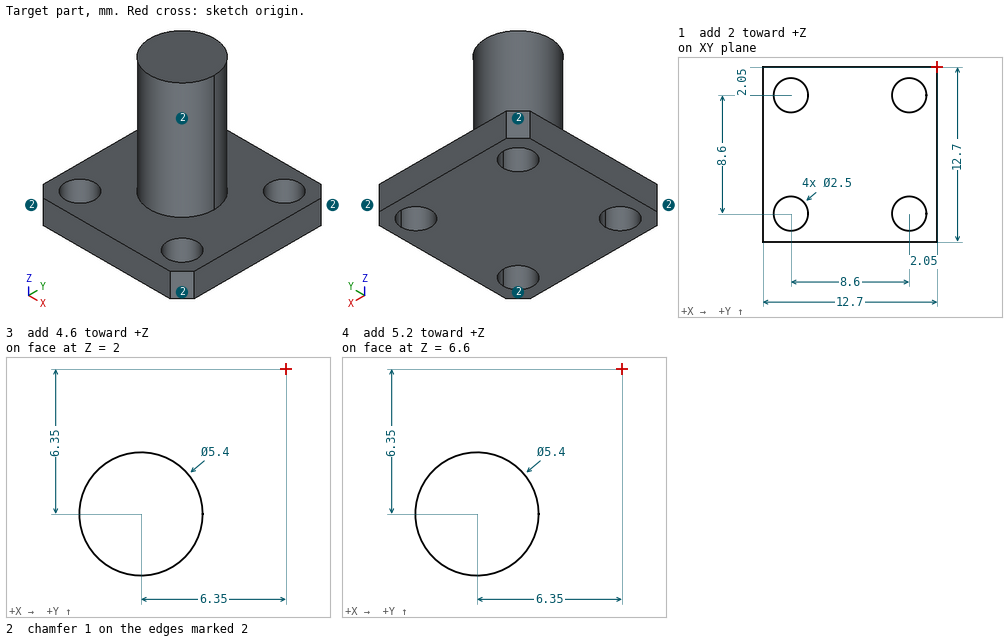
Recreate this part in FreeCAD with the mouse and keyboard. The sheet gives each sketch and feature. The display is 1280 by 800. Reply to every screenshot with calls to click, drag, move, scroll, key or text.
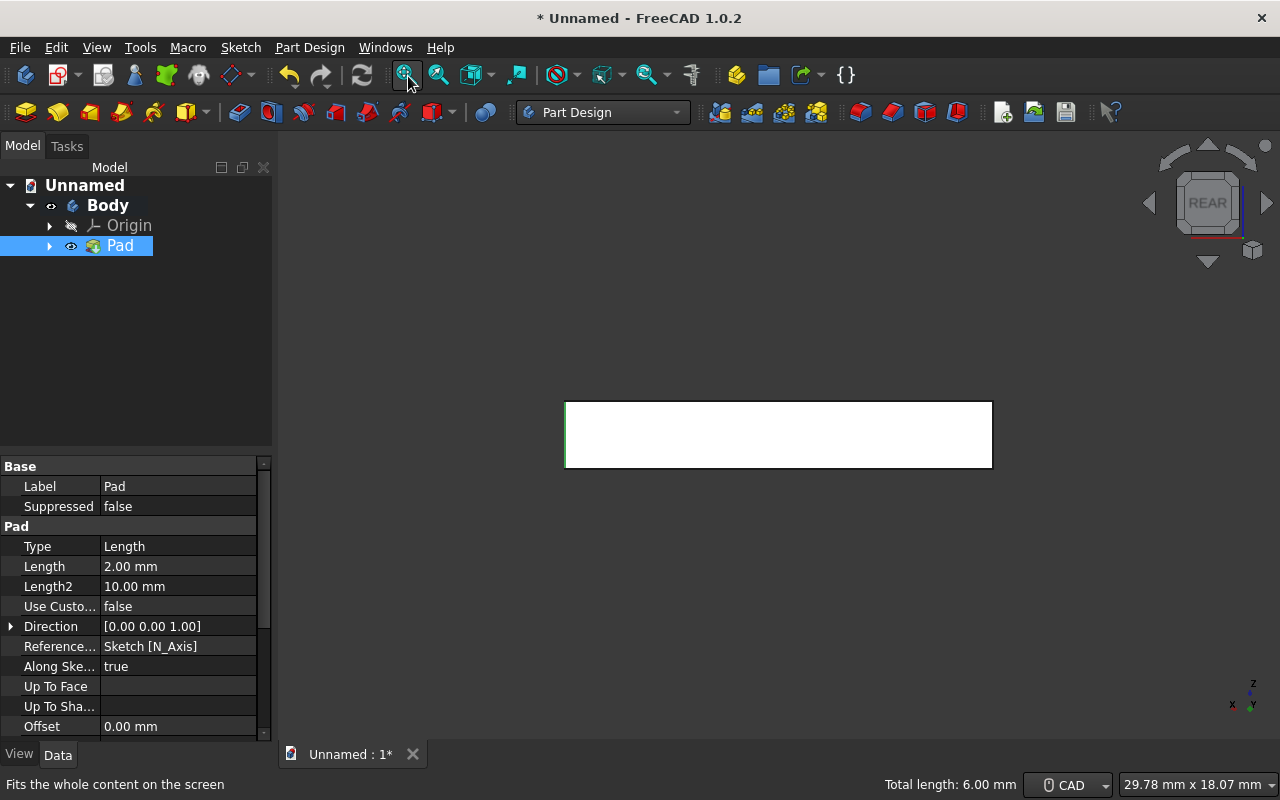
click(993, 434, ctrl)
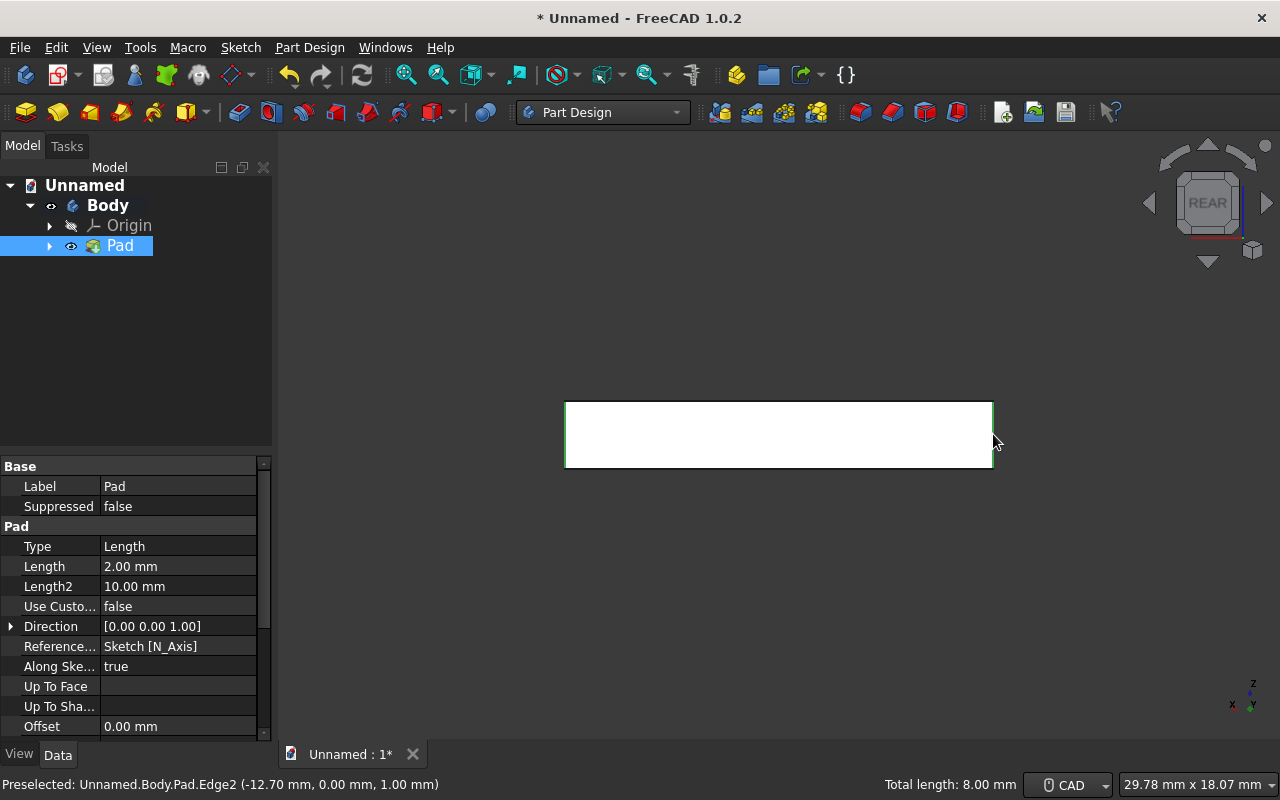
click(894, 112)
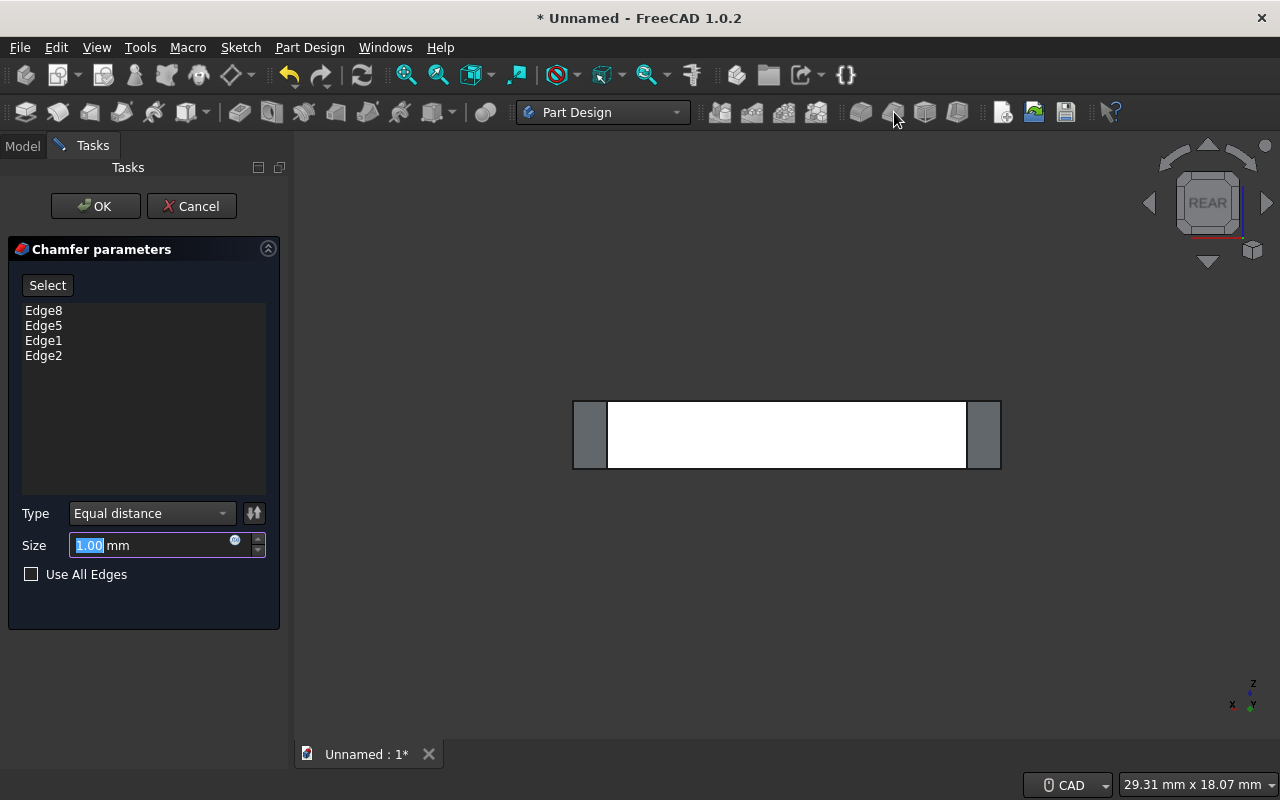
text(1)
key(Tab)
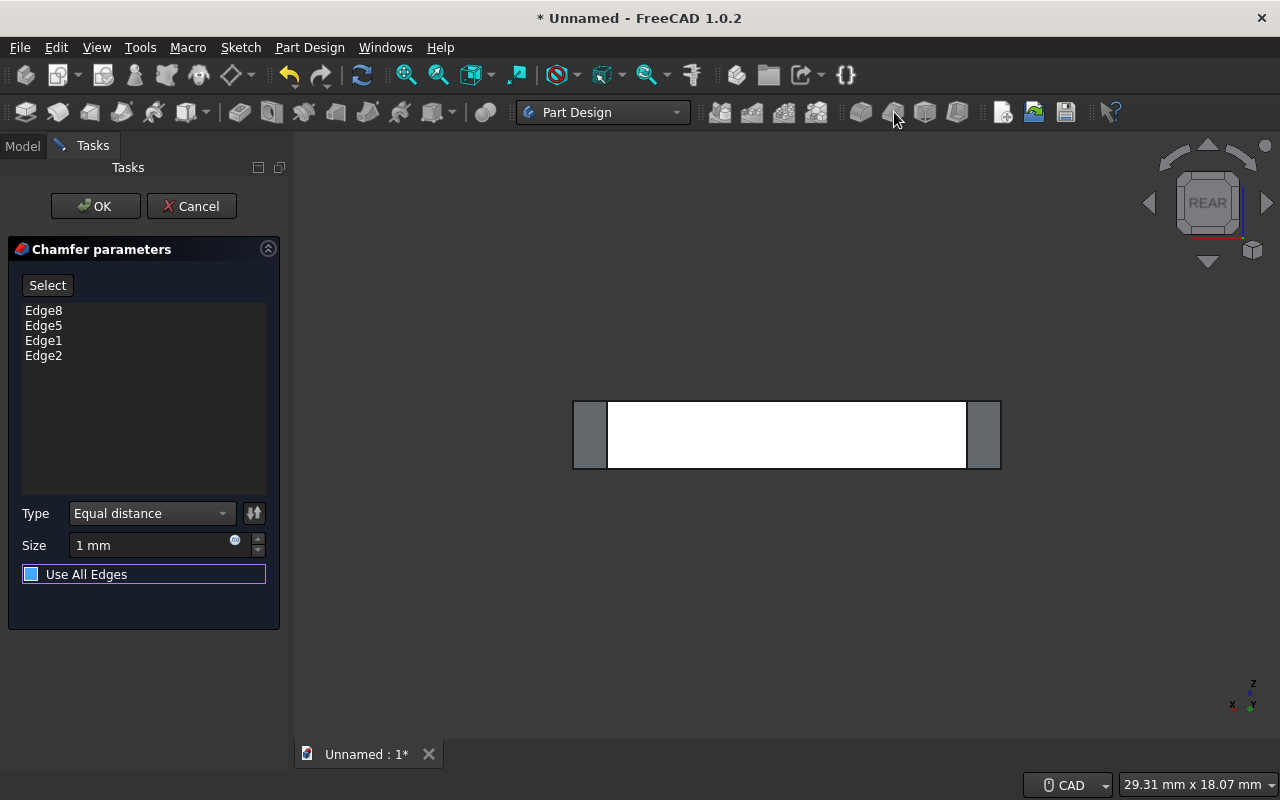
click(96, 206)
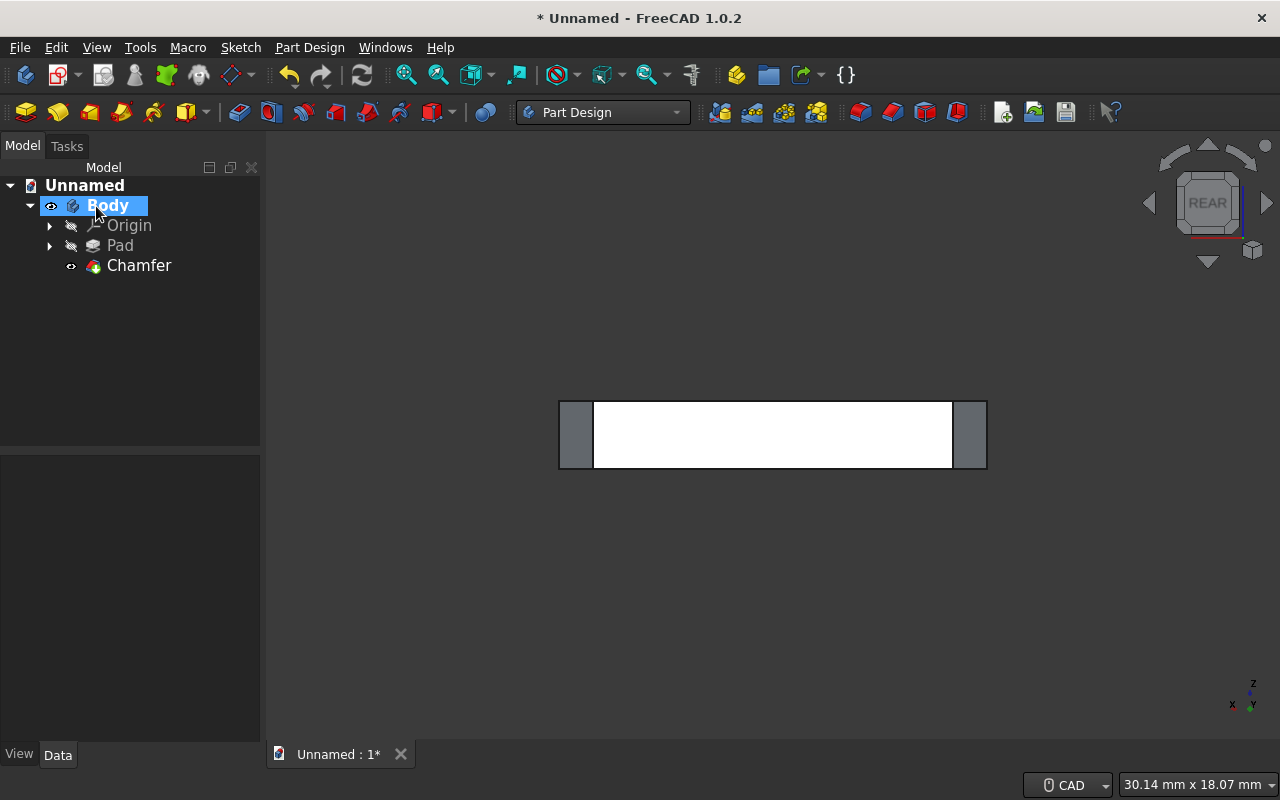
key(v)
key(f)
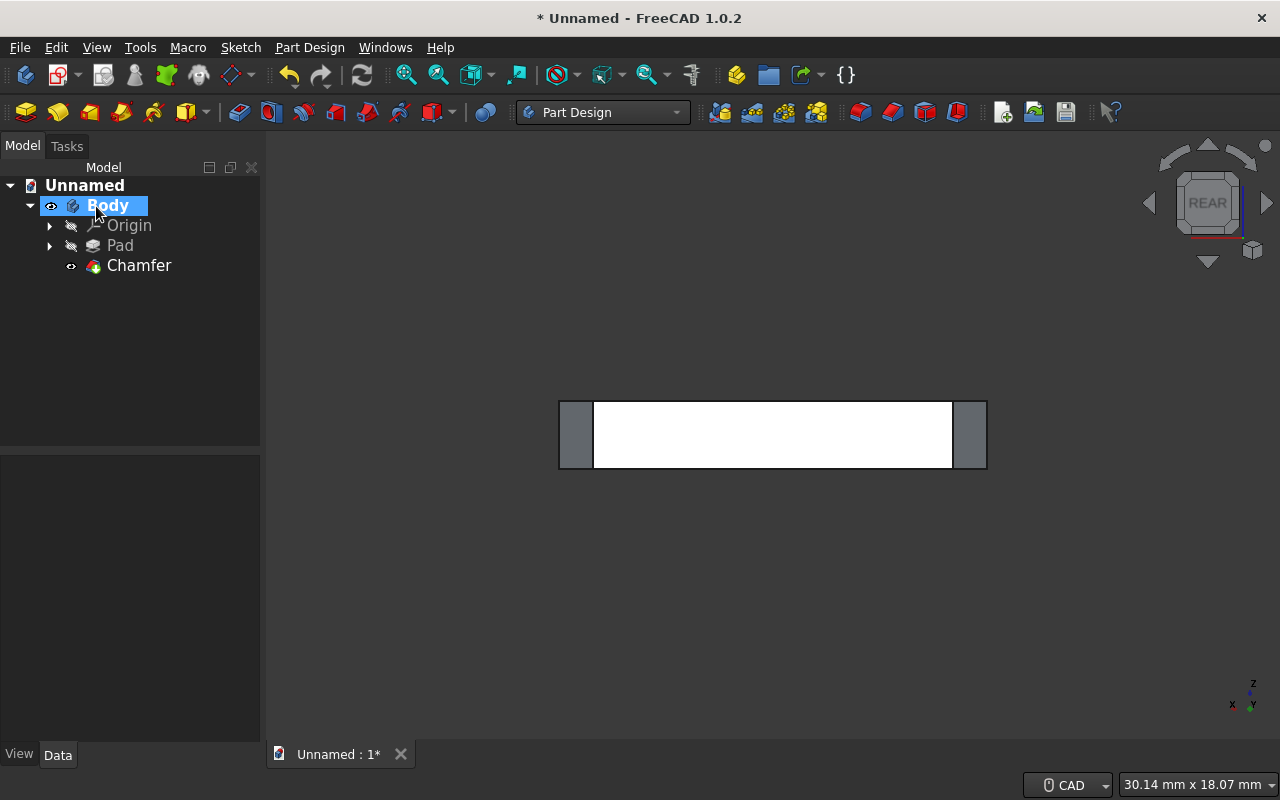
key(0)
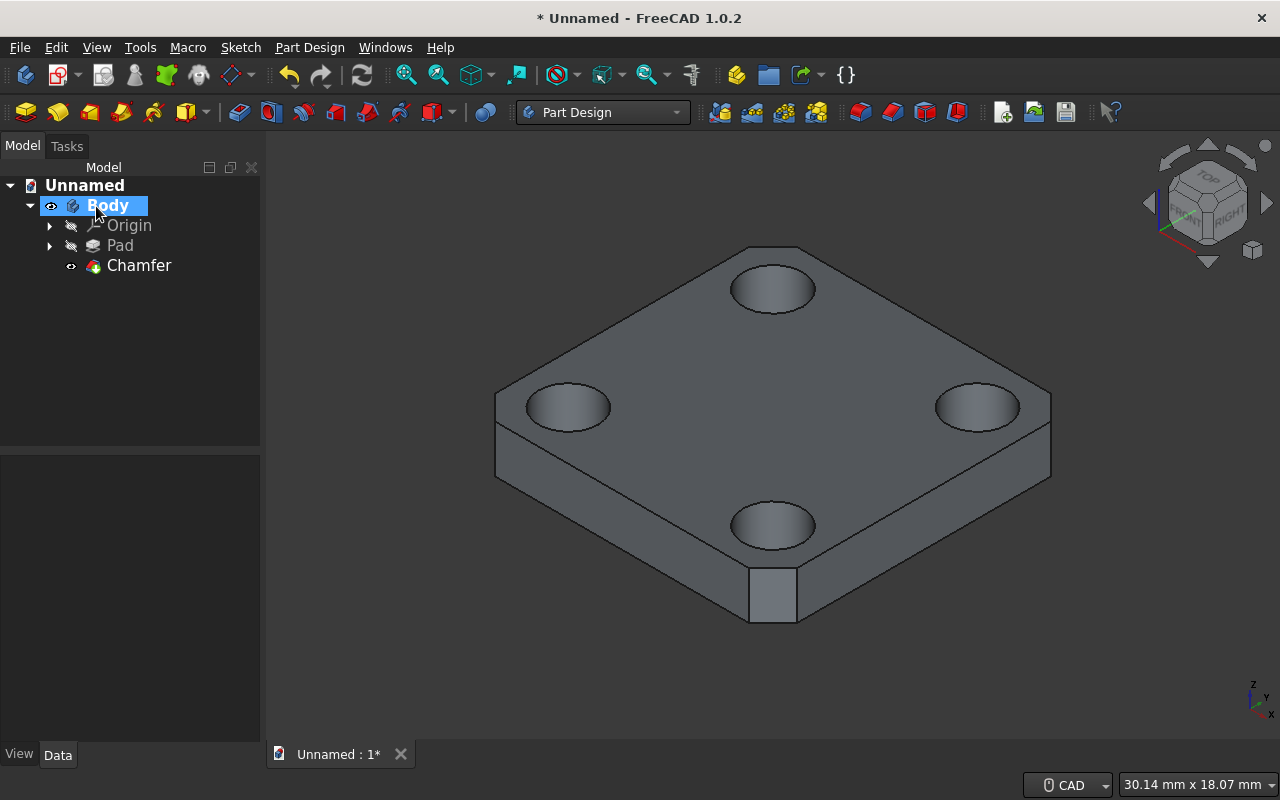
click(773, 407)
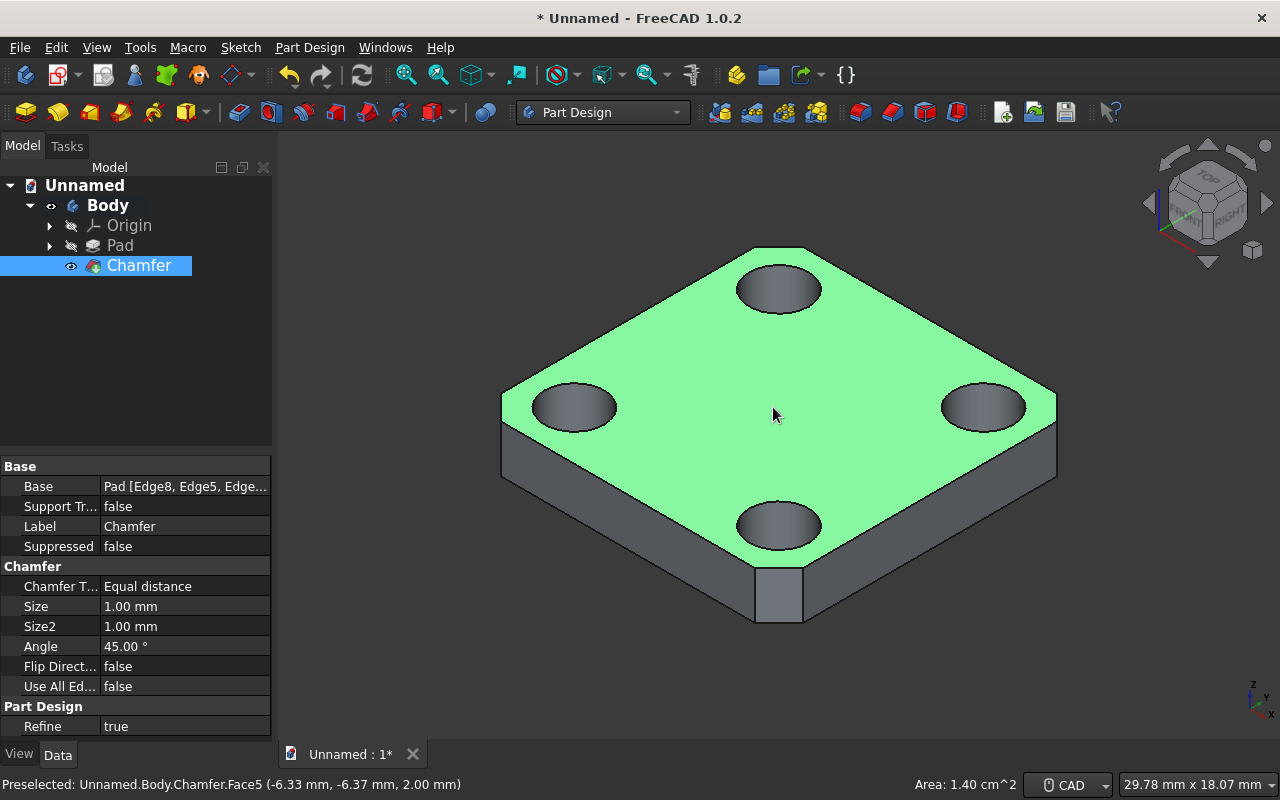
click(58, 76)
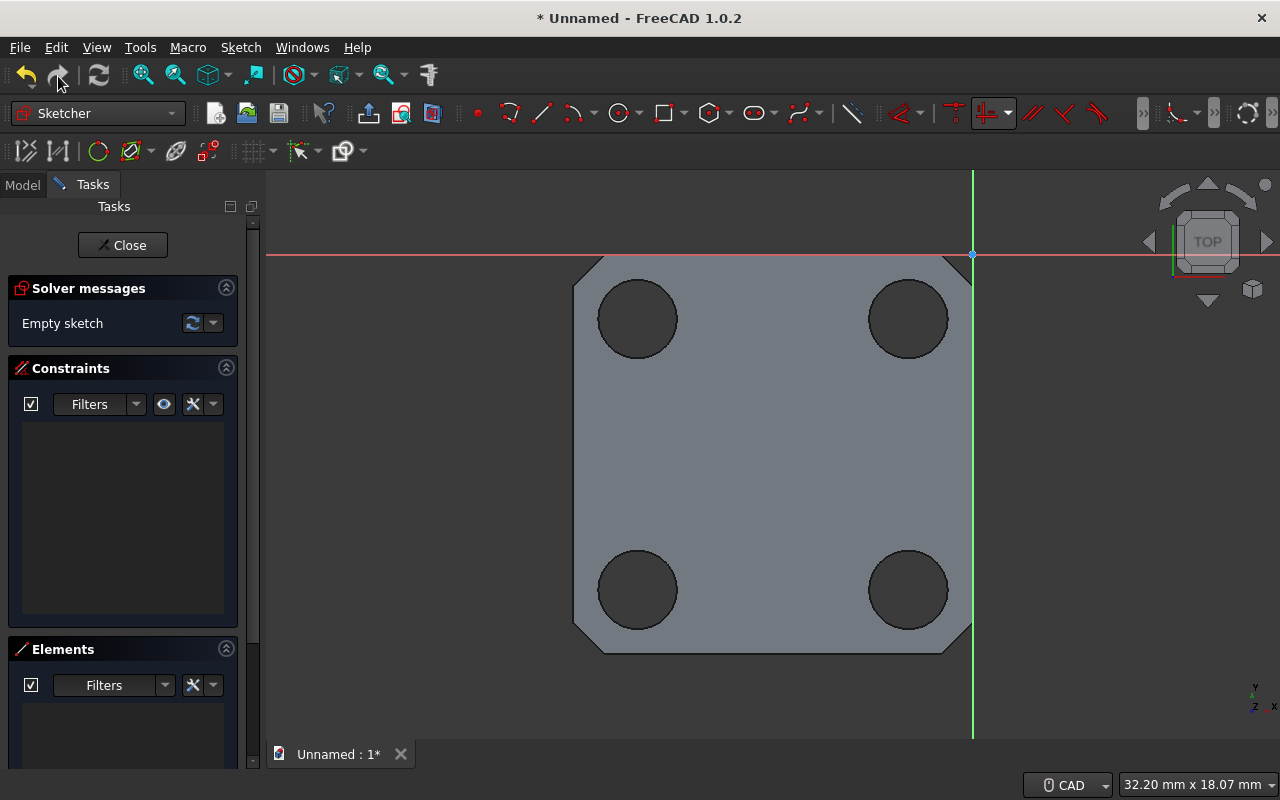
click(620, 114)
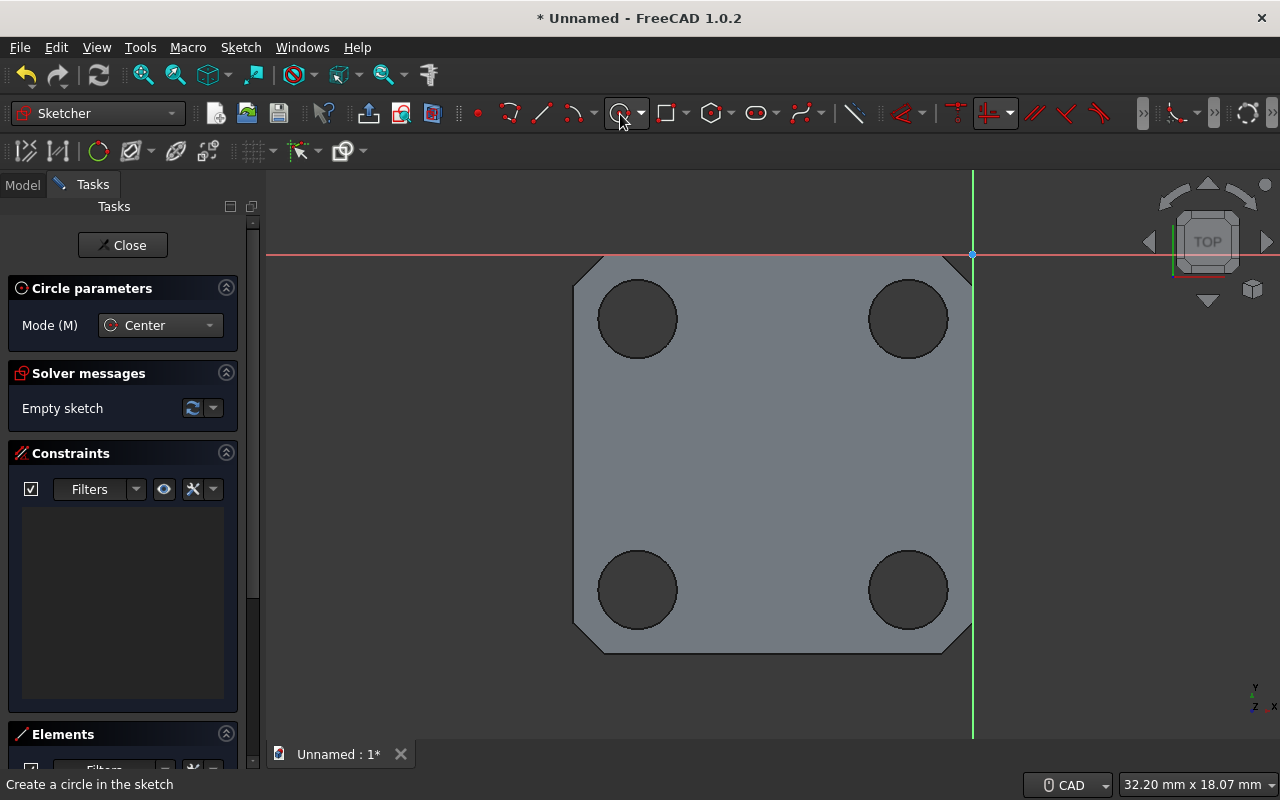
click(773, 454)
move(833, 394)